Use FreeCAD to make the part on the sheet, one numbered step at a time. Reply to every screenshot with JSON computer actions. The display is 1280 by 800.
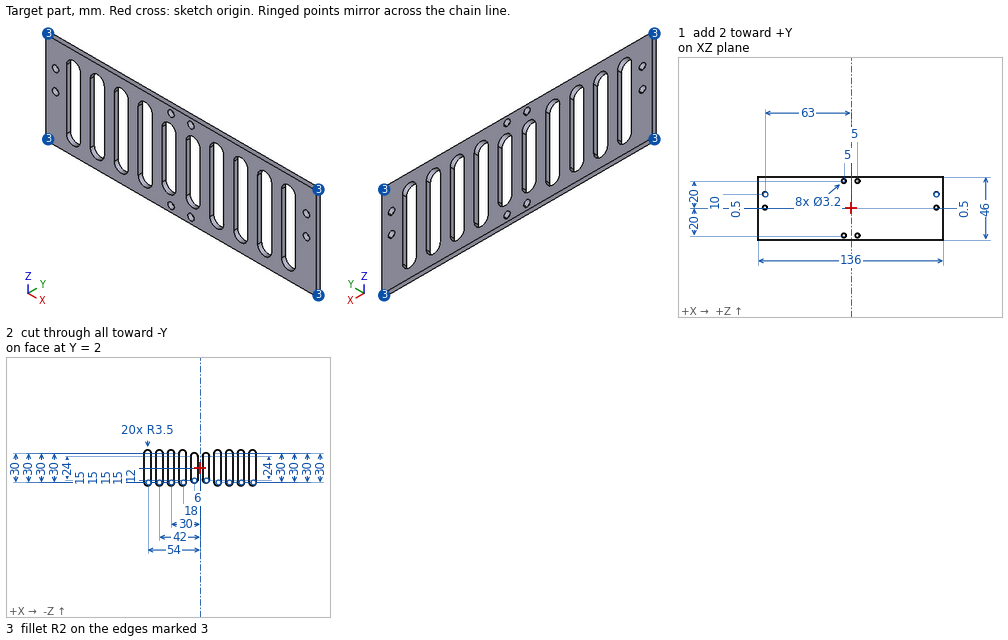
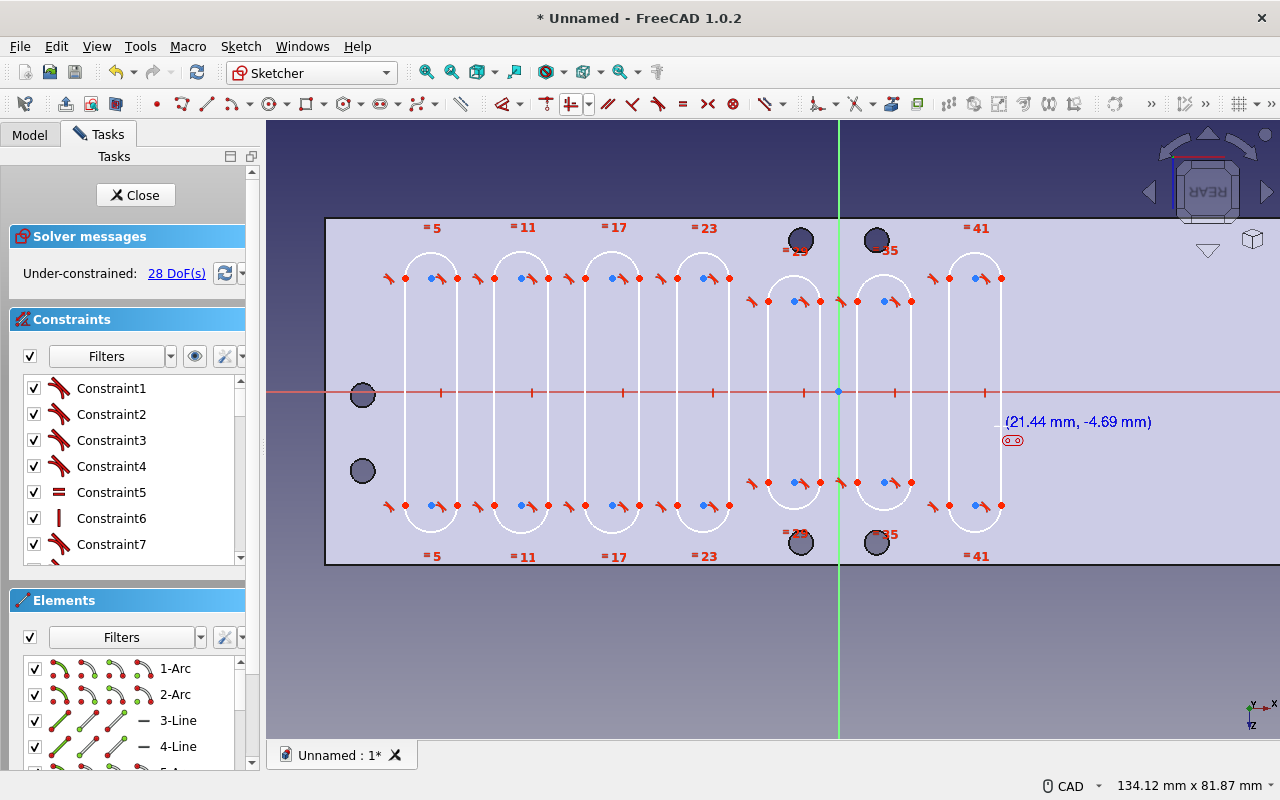
{"action": "left_click", "coordinate": [1066, 505]}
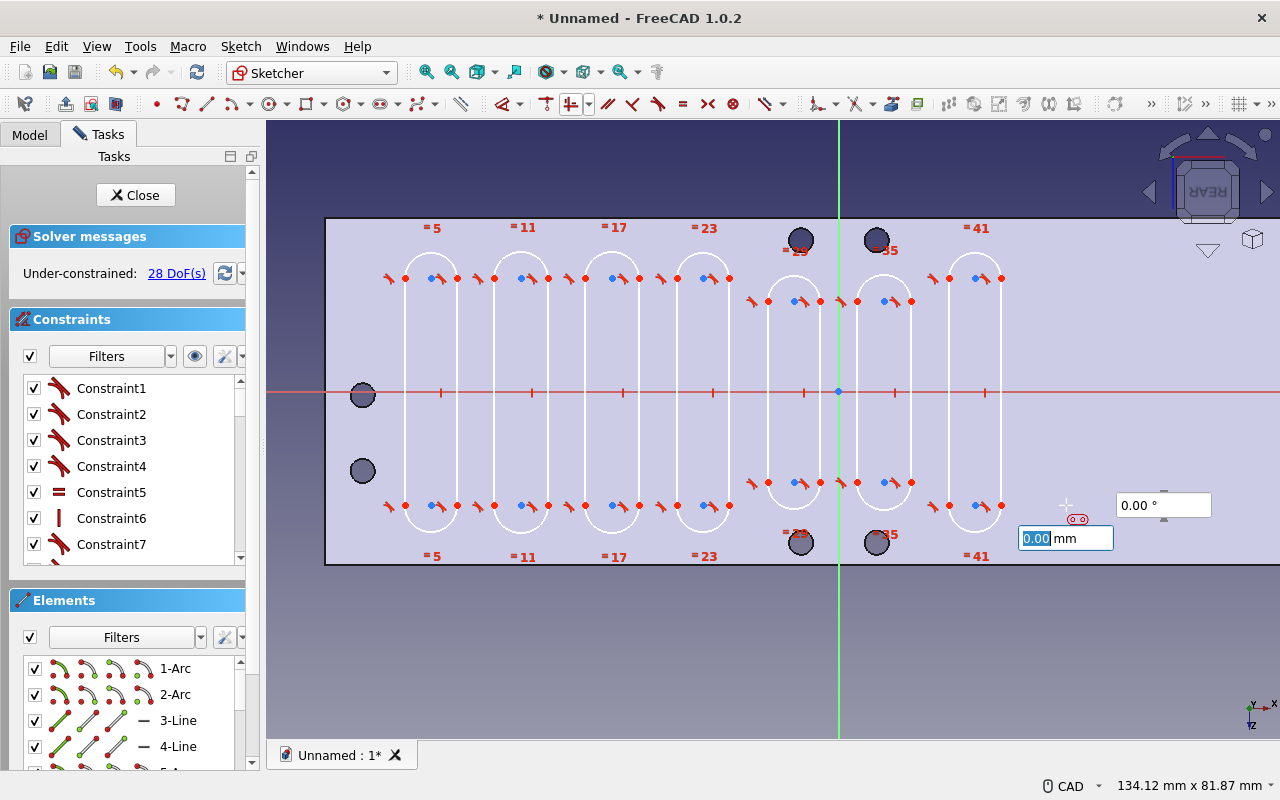
{"action": "left_click", "coordinate": [1066, 278]}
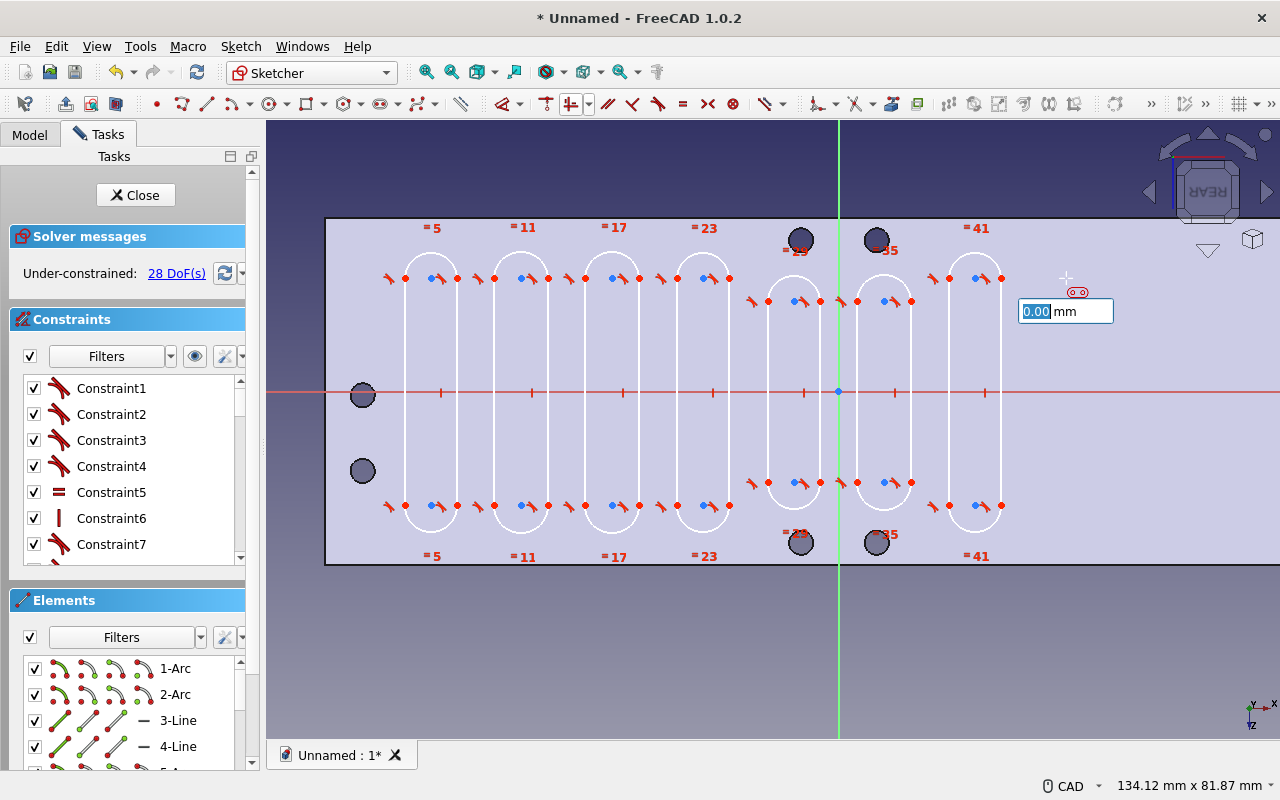
{"action": "left_click", "coordinate": [1092, 426]}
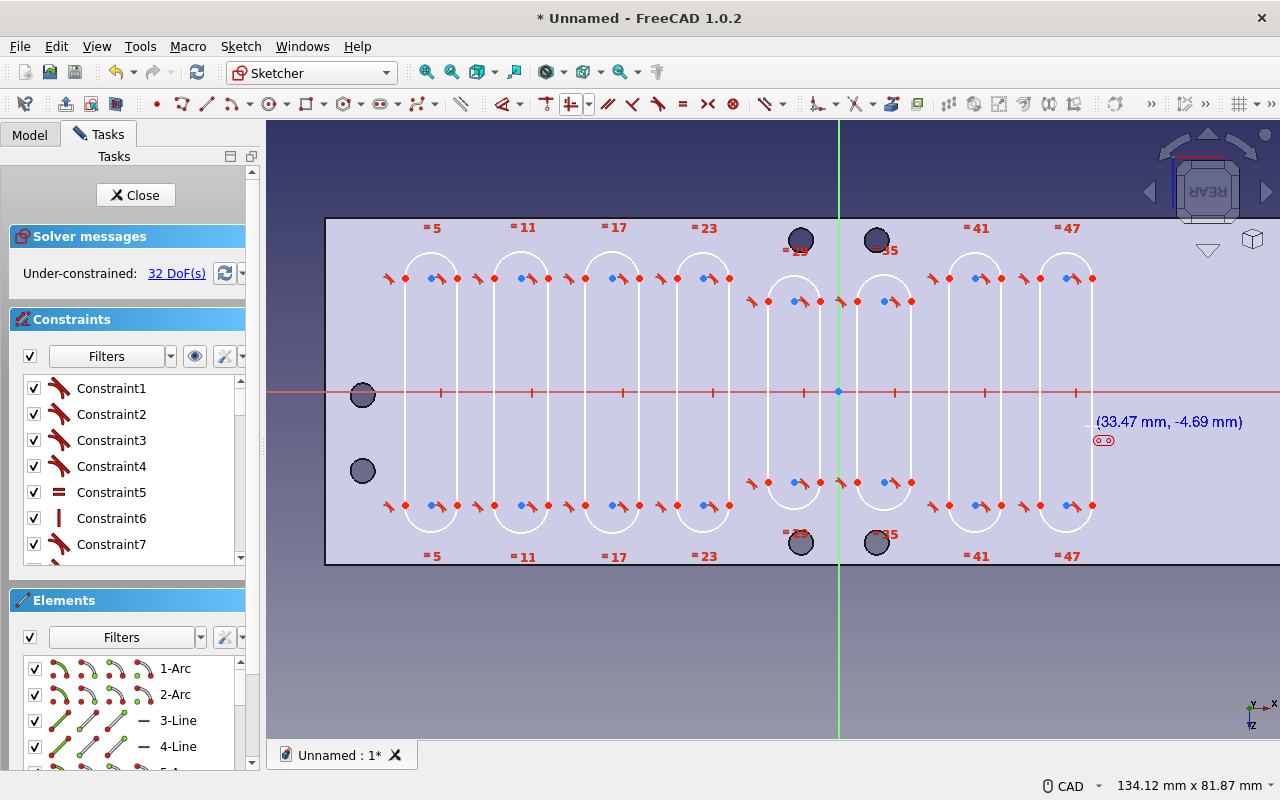
{"action": "scroll", "coordinate": [431, 507], "scroll_direction": "down", "scroll_amount": 2}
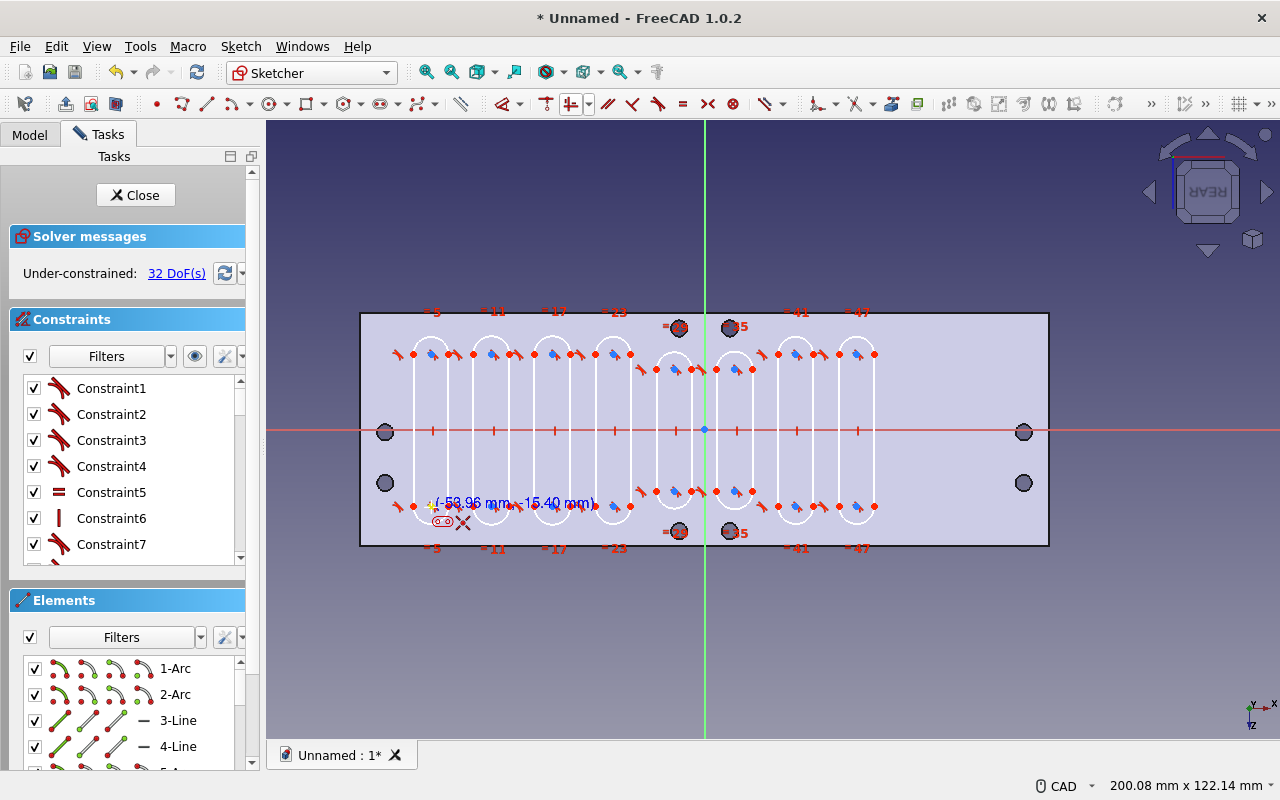
{"action": "scroll", "coordinate": [917, 506], "scroll_direction": "up", "scroll_amount": 2}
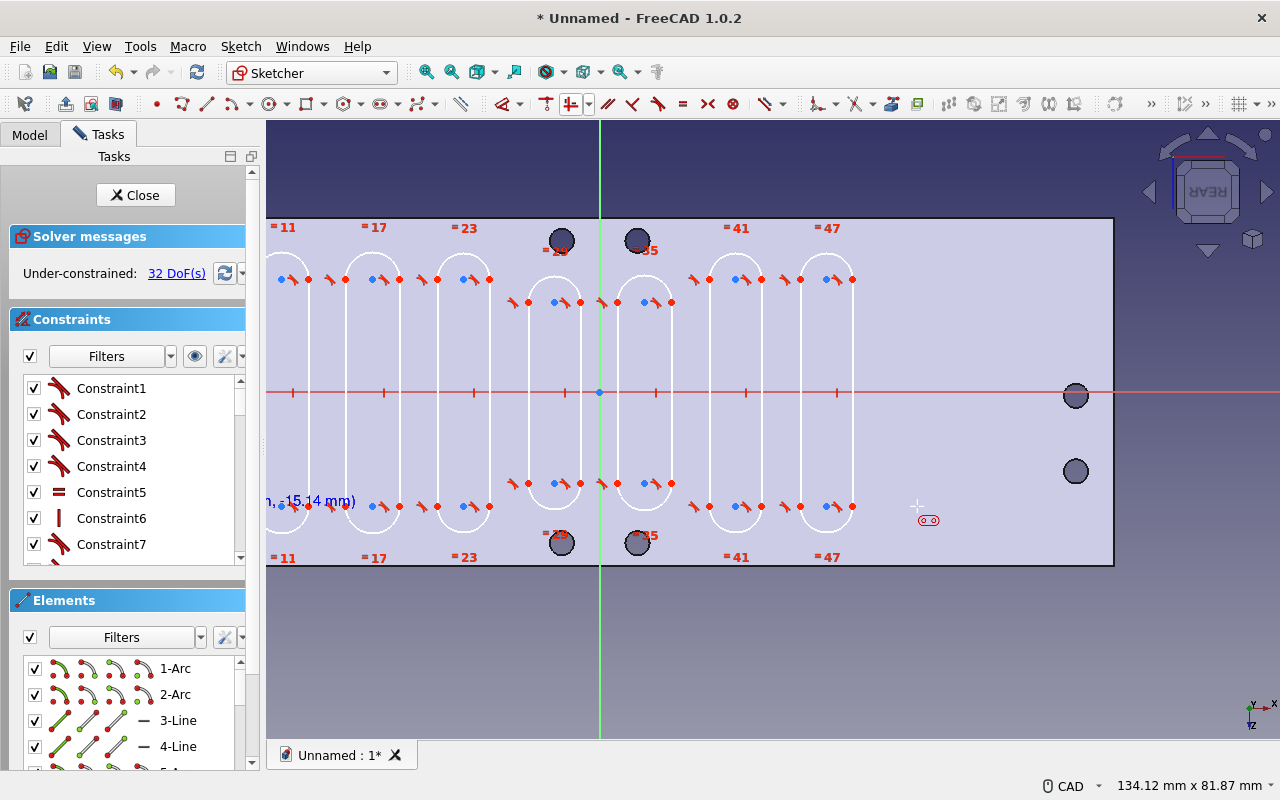
{"action": "left_click", "coordinate": [917, 505]}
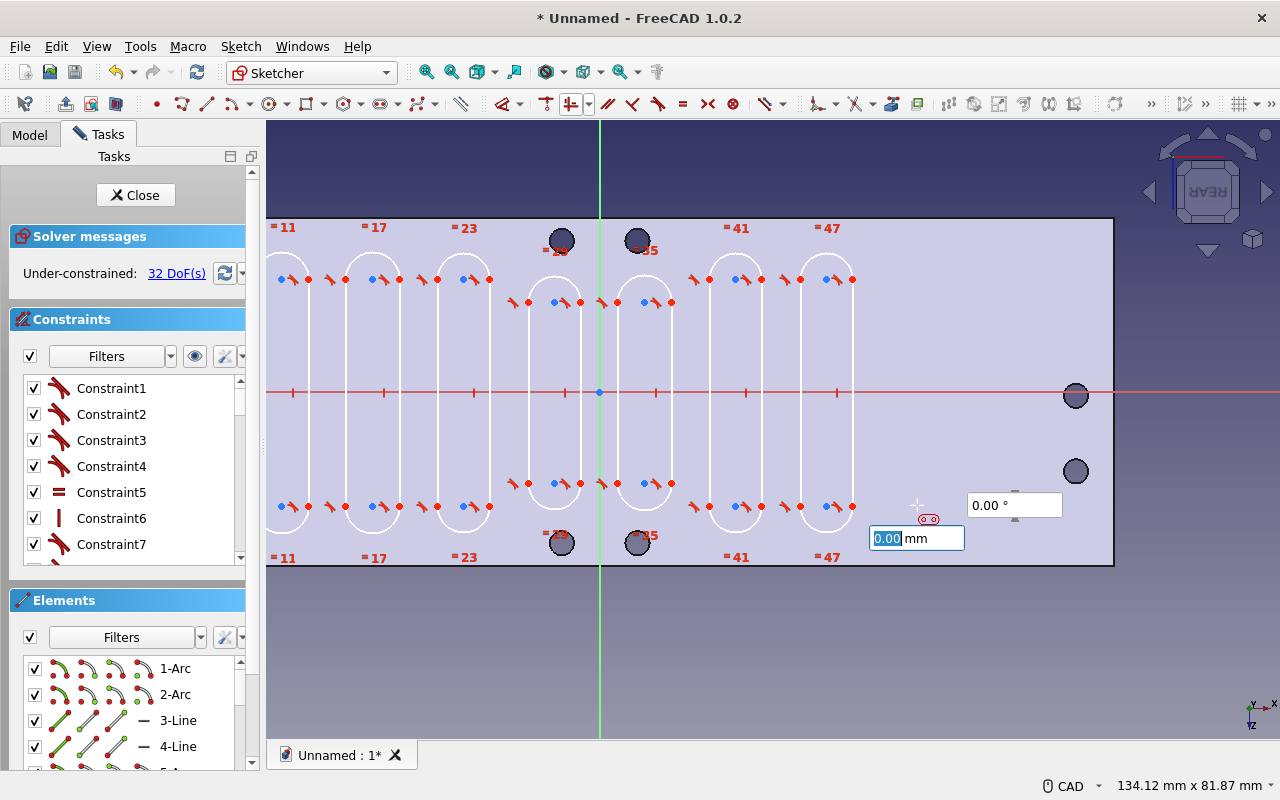
{"action": "left_click", "coordinate": [917, 279]}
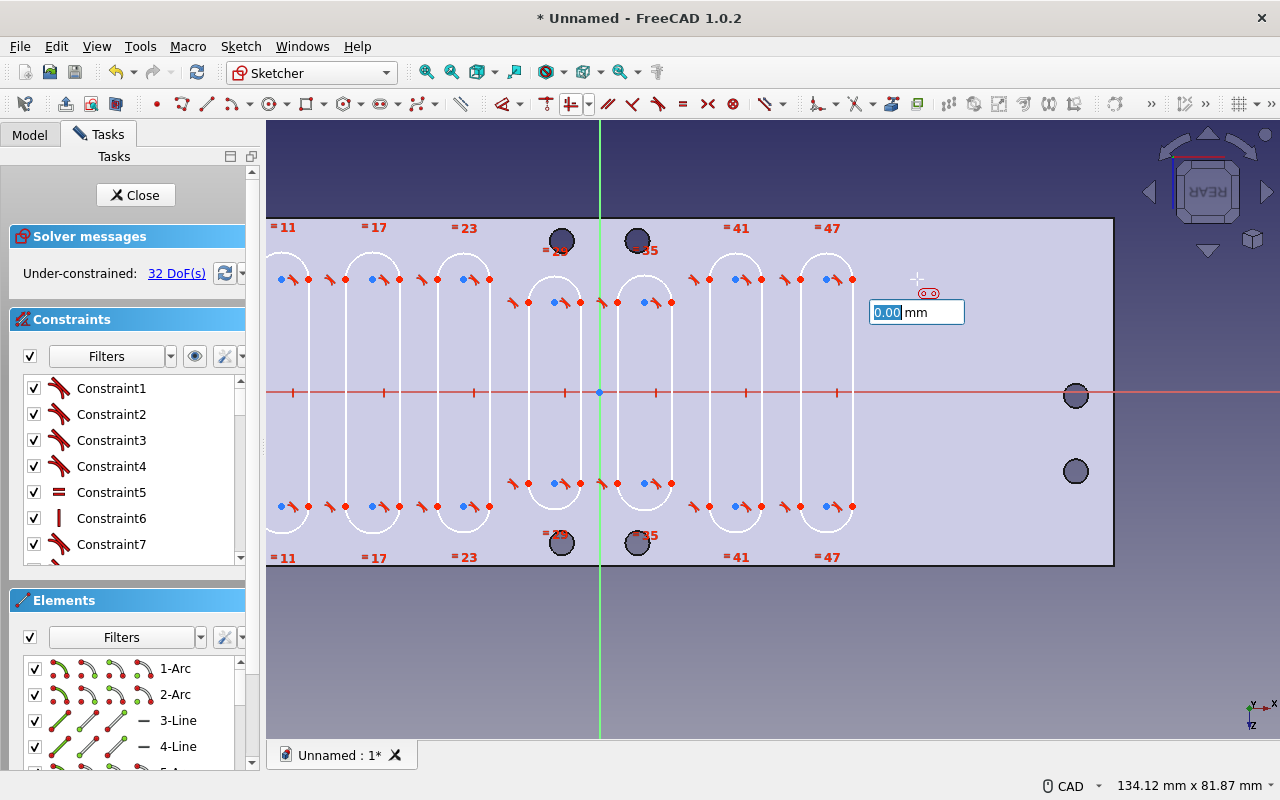
{"action": "left_click", "coordinate": [944, 426]}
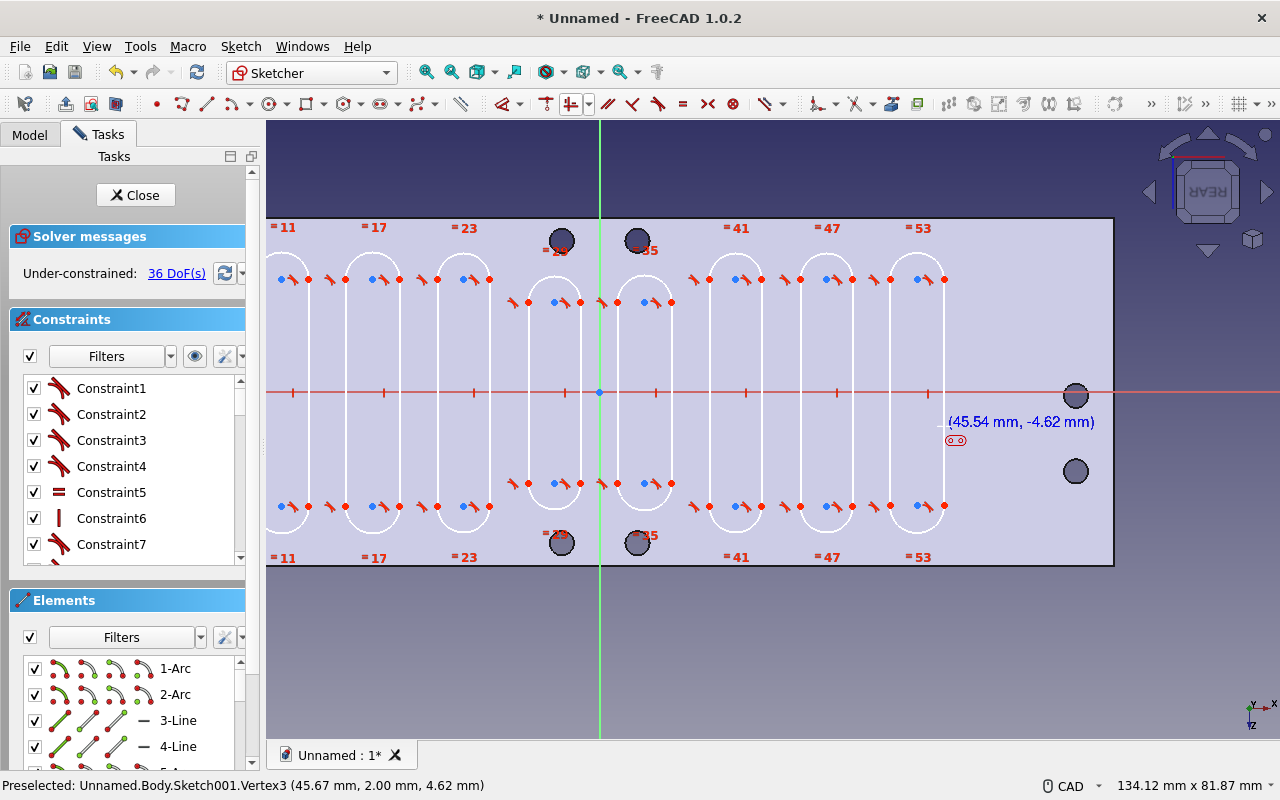
{"action": "left_click", "coordinate": [1008, 505]}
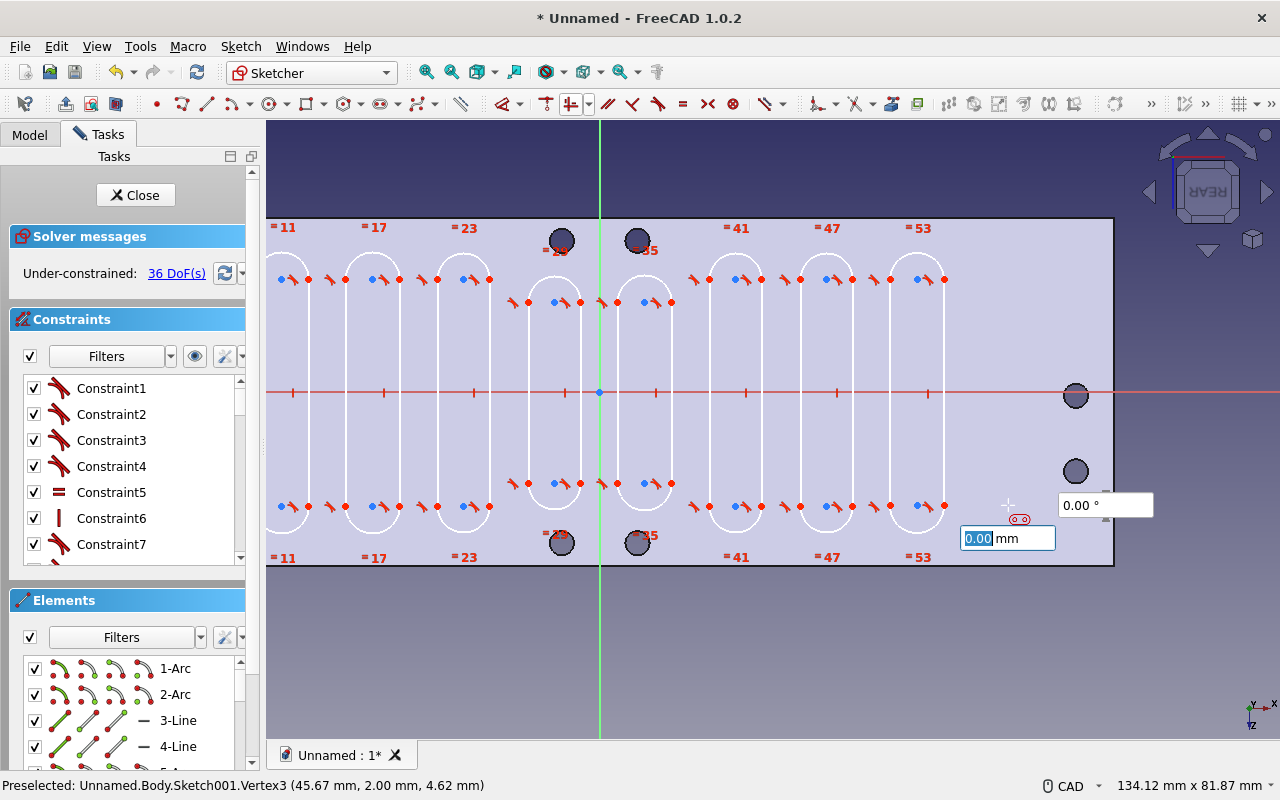
{"action": "left_click", "coordinate": [1008, 279]}